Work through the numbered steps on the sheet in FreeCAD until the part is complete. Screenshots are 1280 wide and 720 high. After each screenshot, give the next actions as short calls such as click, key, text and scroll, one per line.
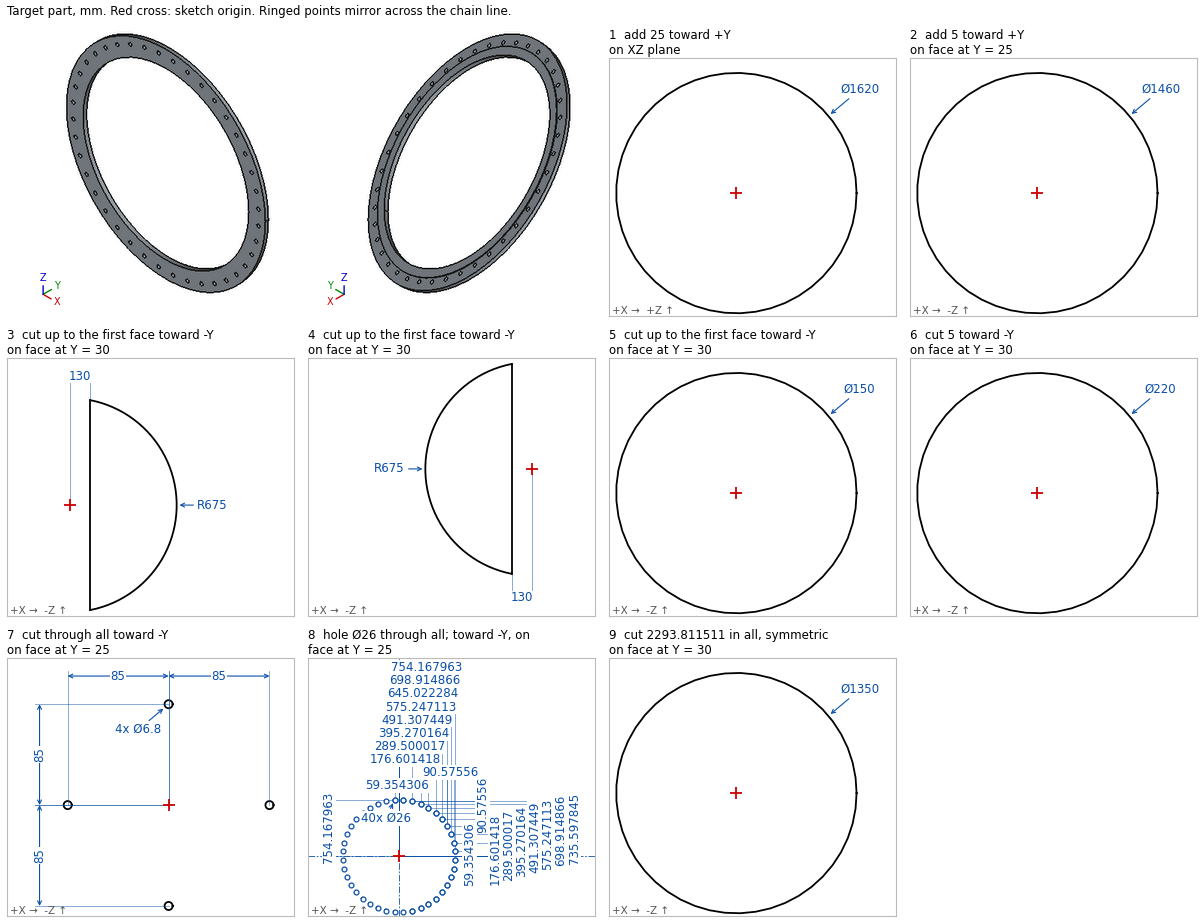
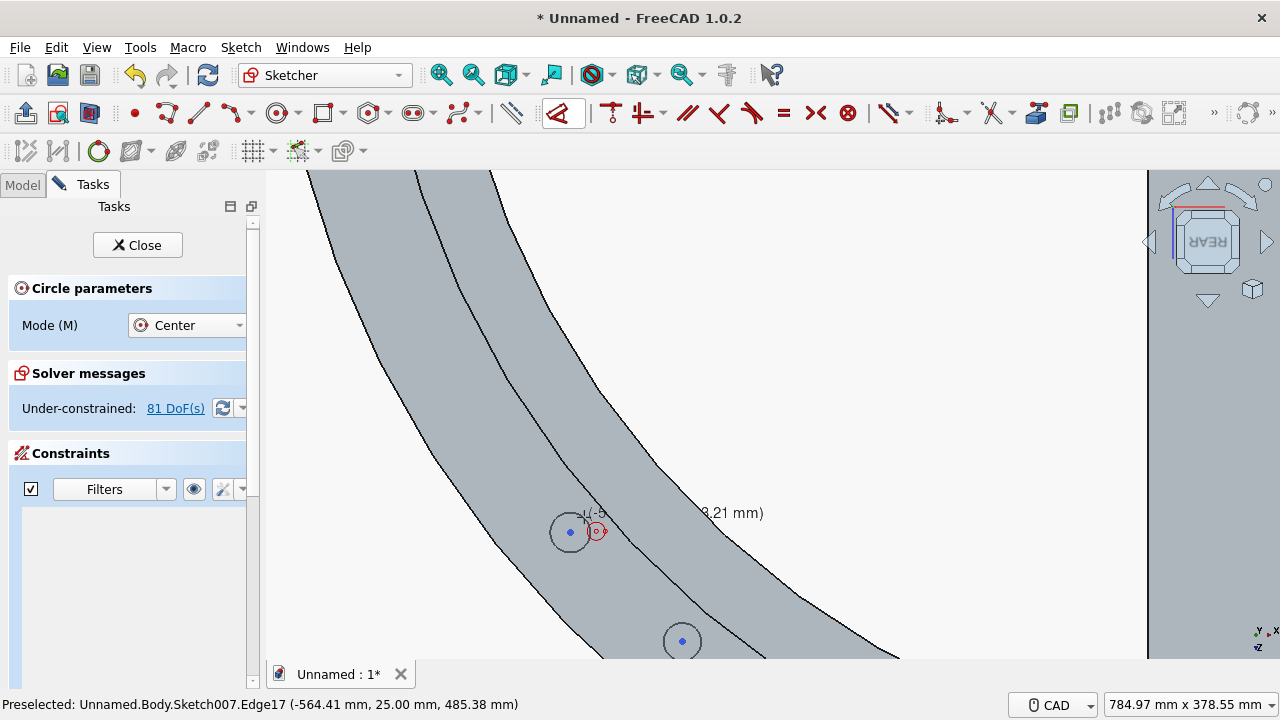
scroll(482, 404, up, 2)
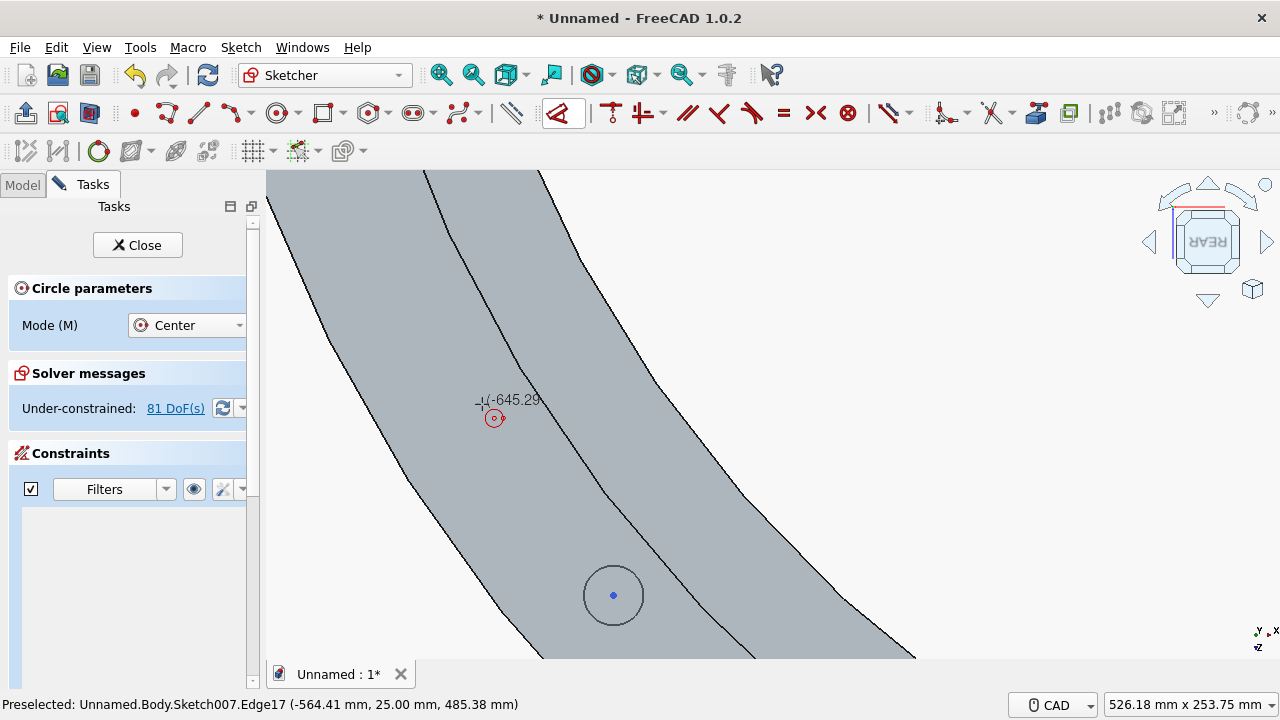
scroll(577, 511, down, 11)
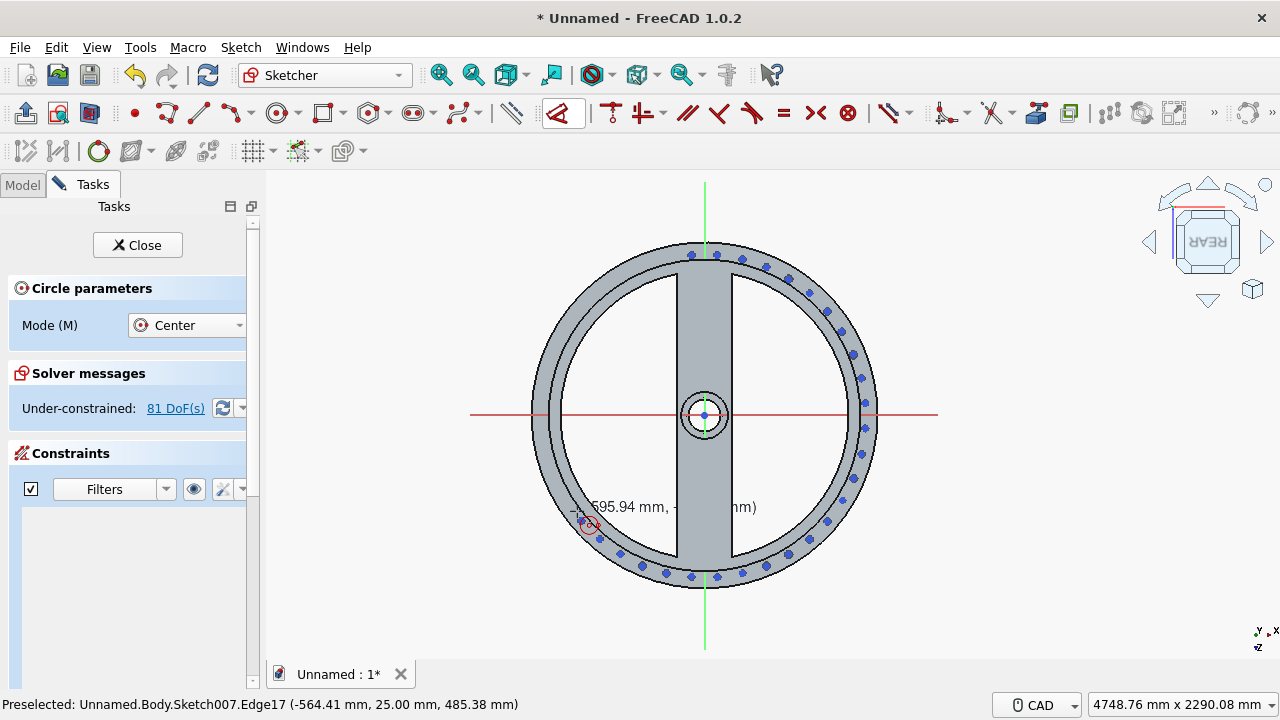
click(567, 500)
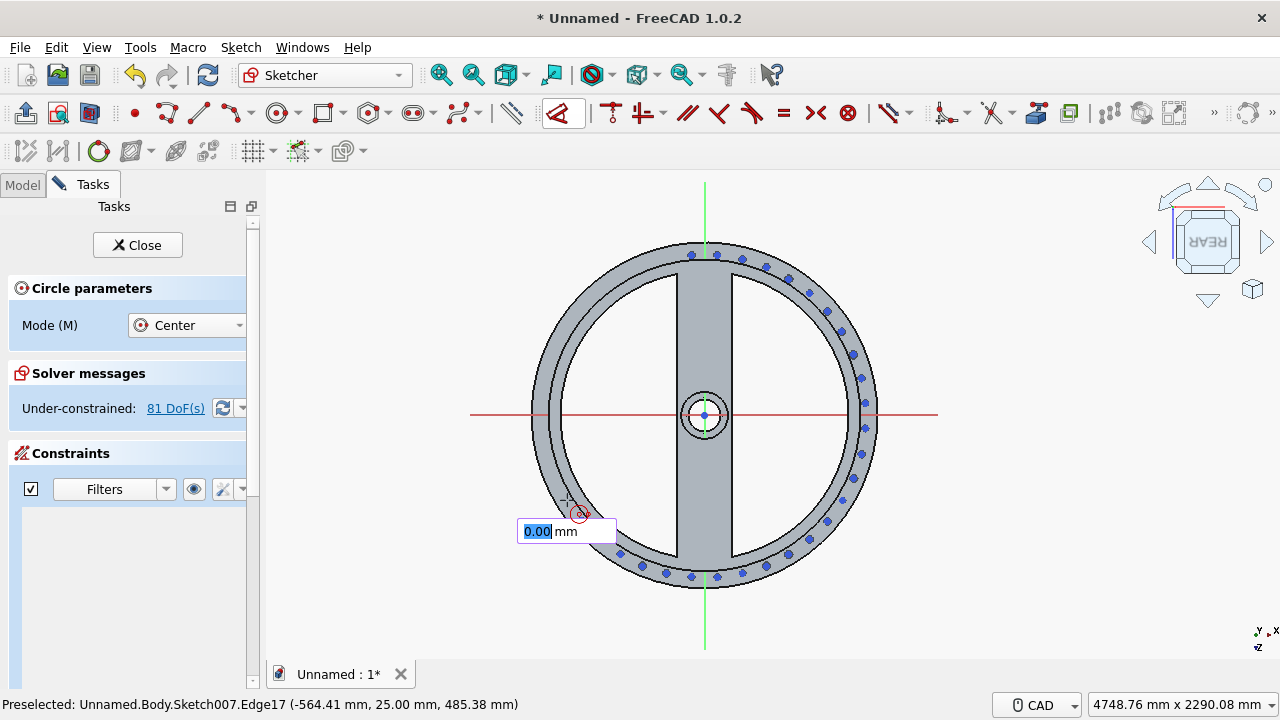
scroll(569, 498, up, 9)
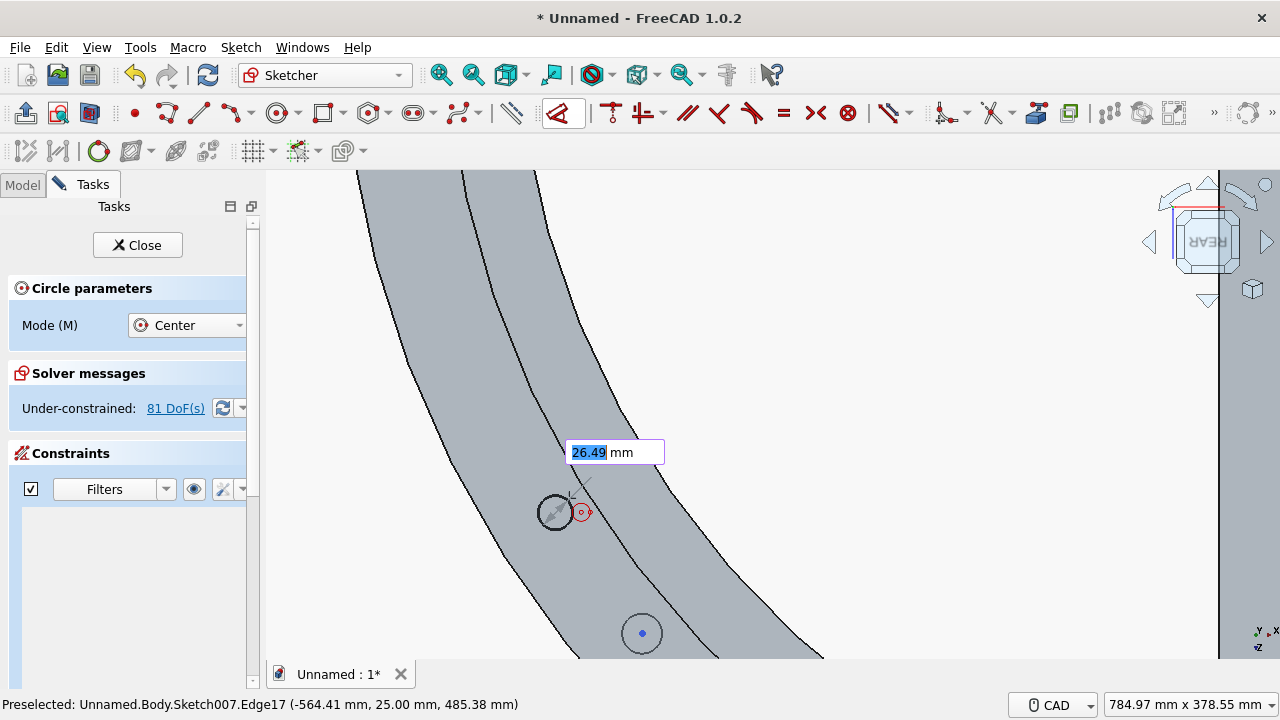
click(566, 494)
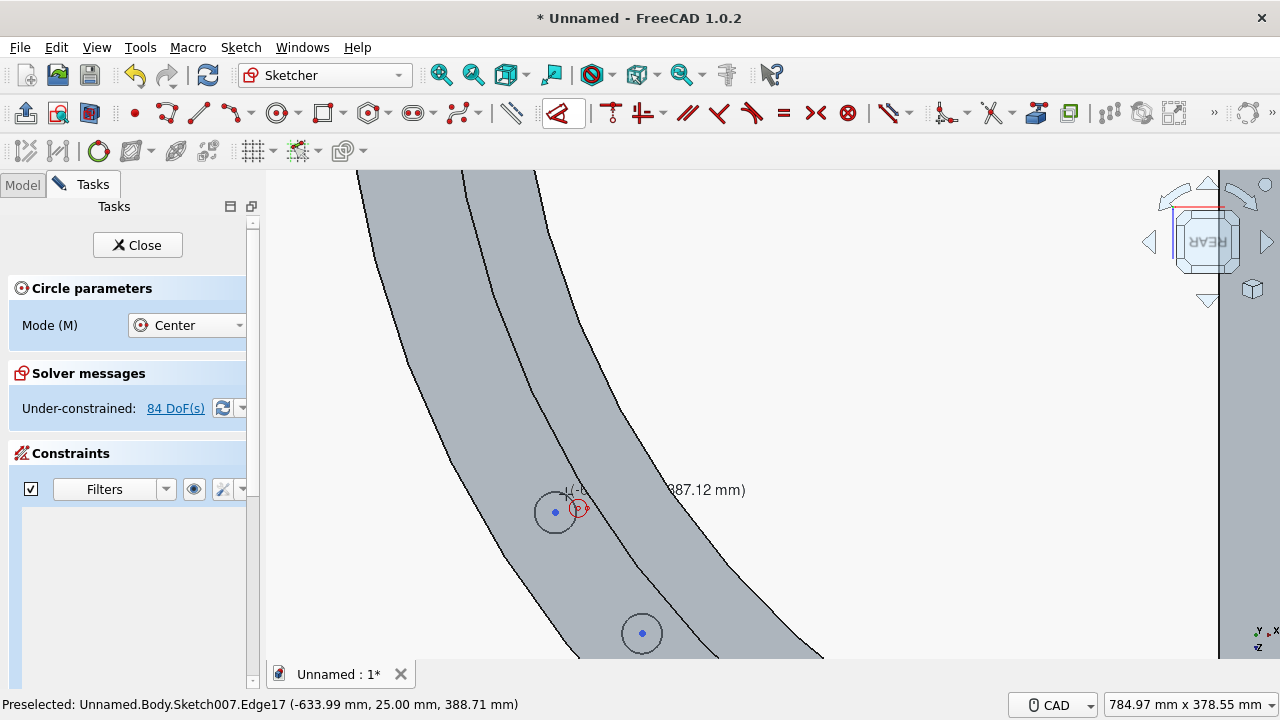
scroll(485, 369, up, 2)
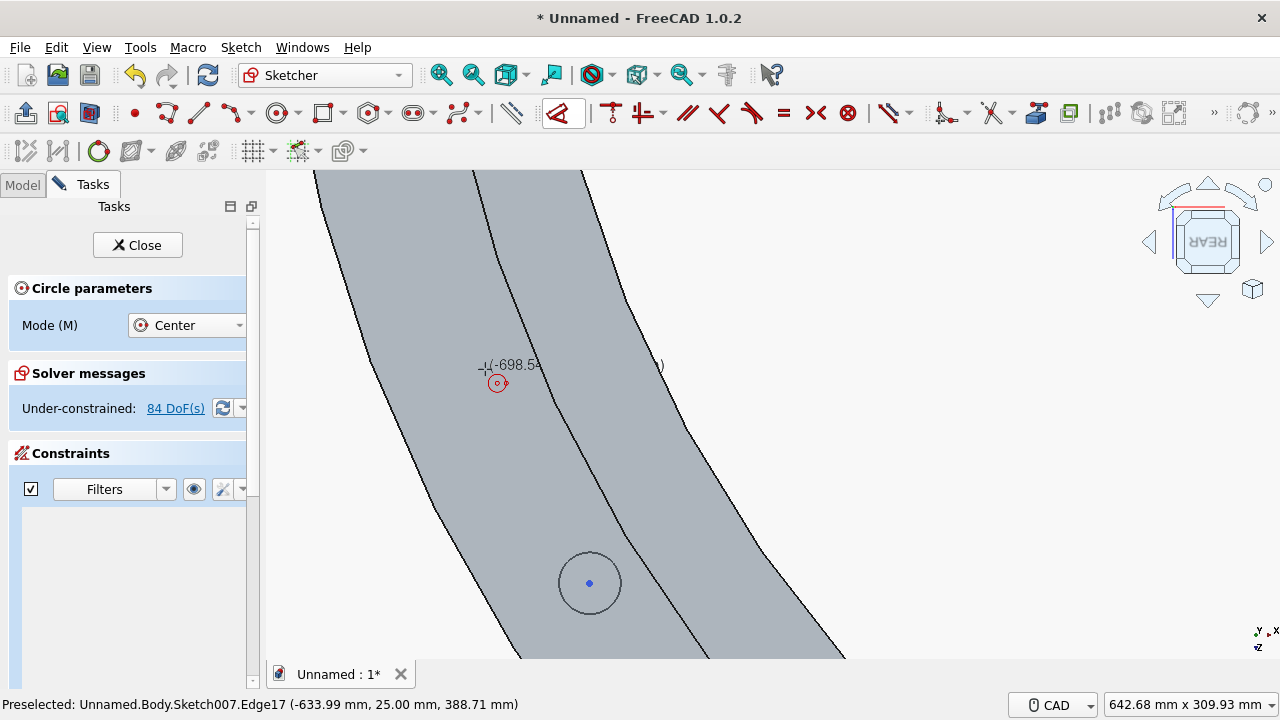
scroll(564, 490, down, 11)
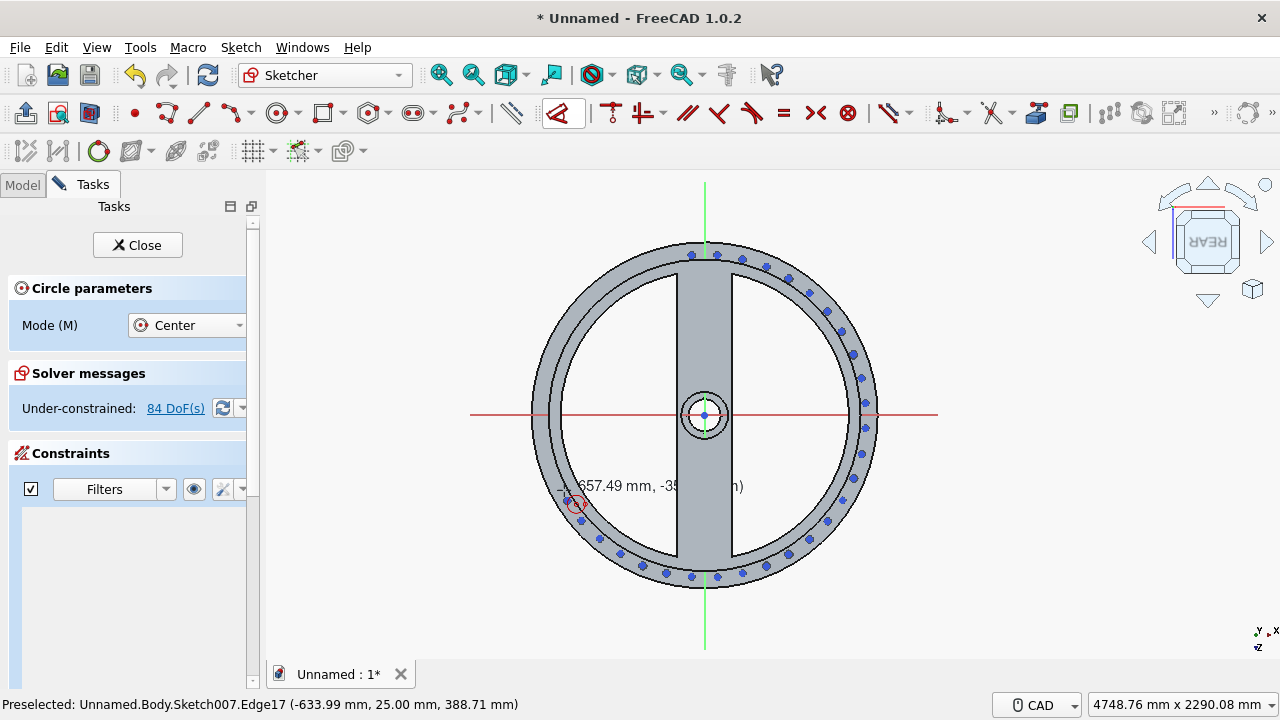
click(555, 477)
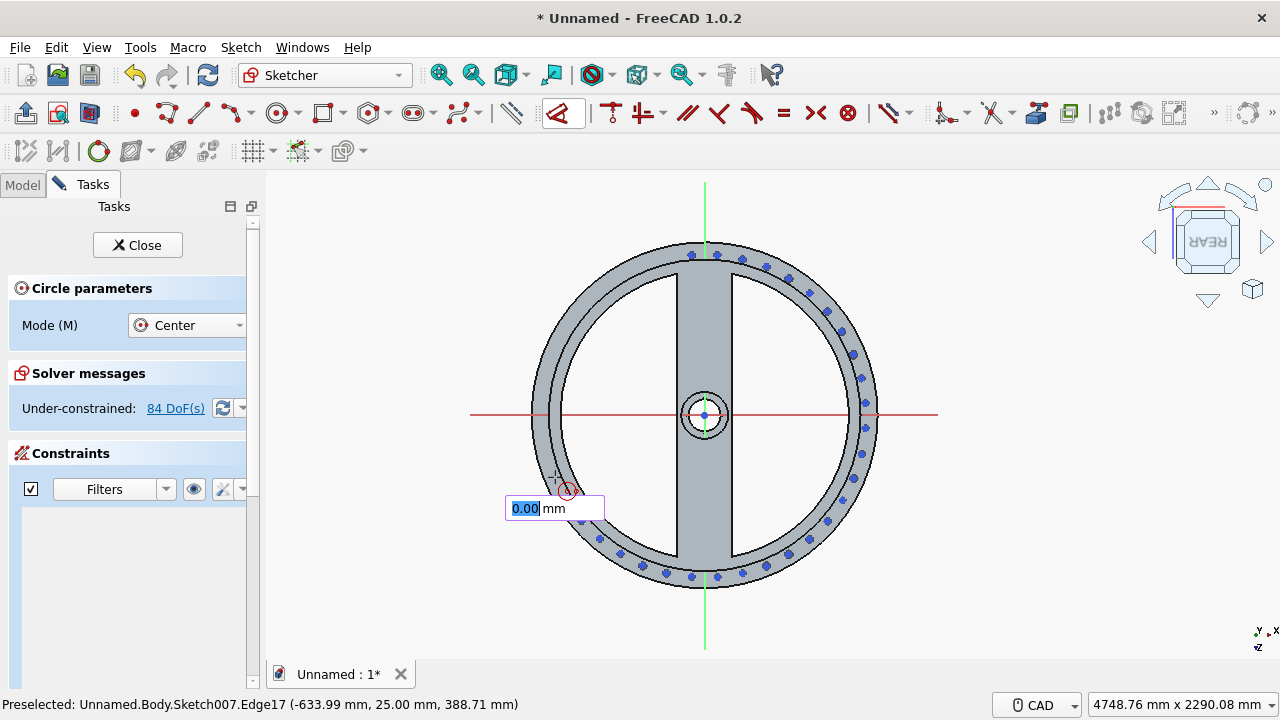
scroll(557, 475, up, 9)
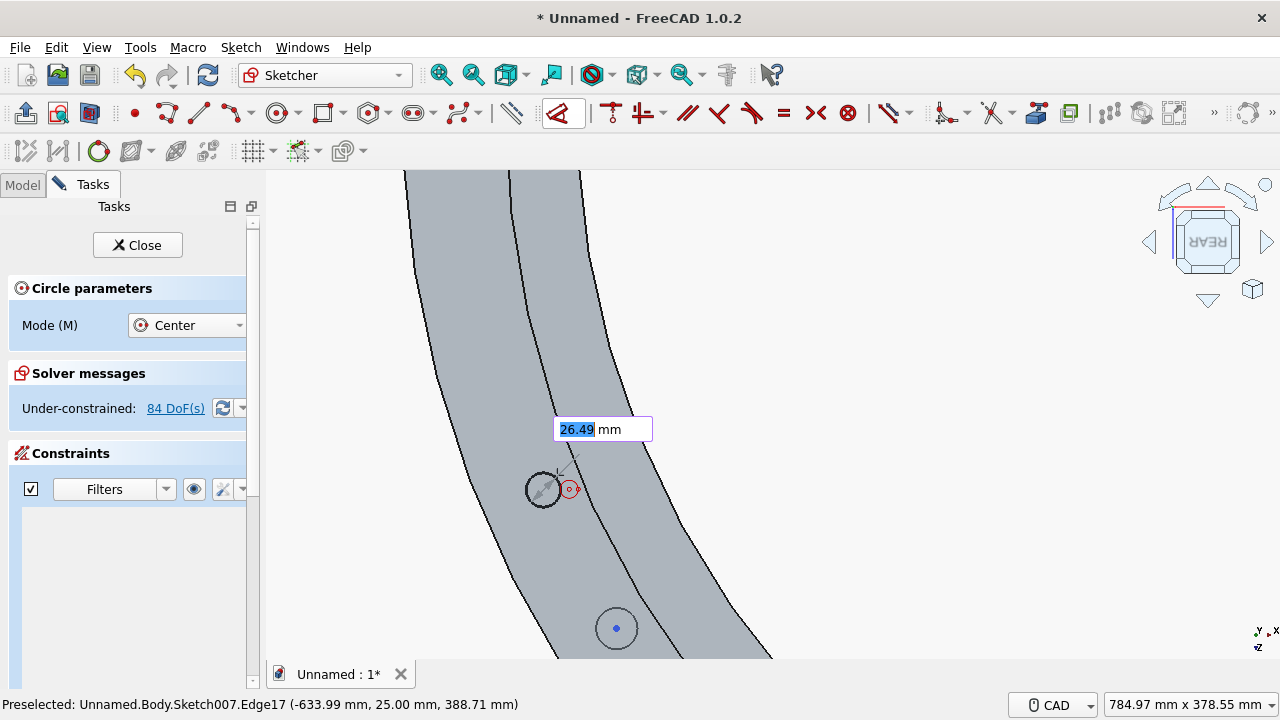
click(558, 473)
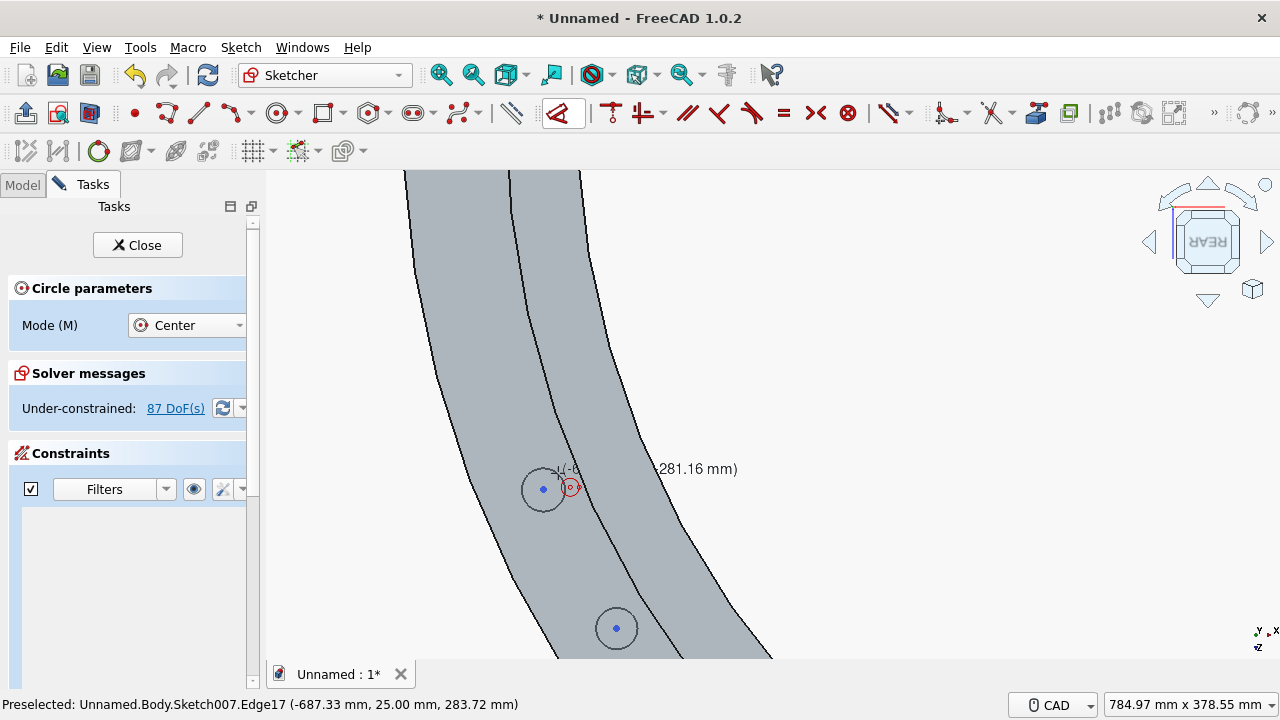
scroll(499, 339, up, 2)